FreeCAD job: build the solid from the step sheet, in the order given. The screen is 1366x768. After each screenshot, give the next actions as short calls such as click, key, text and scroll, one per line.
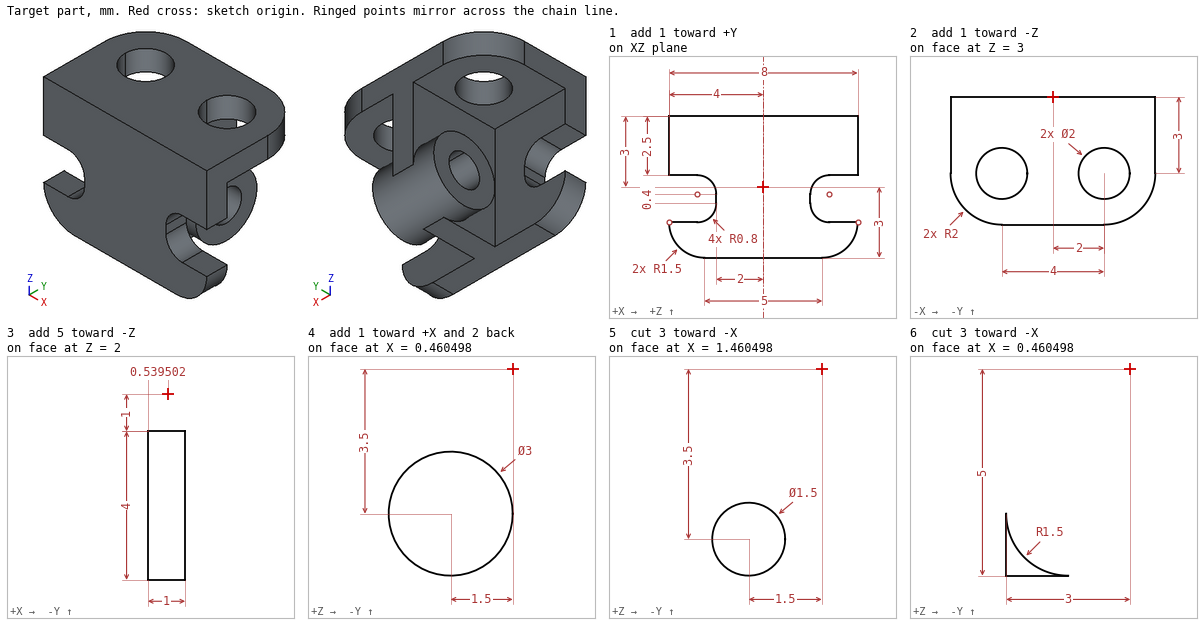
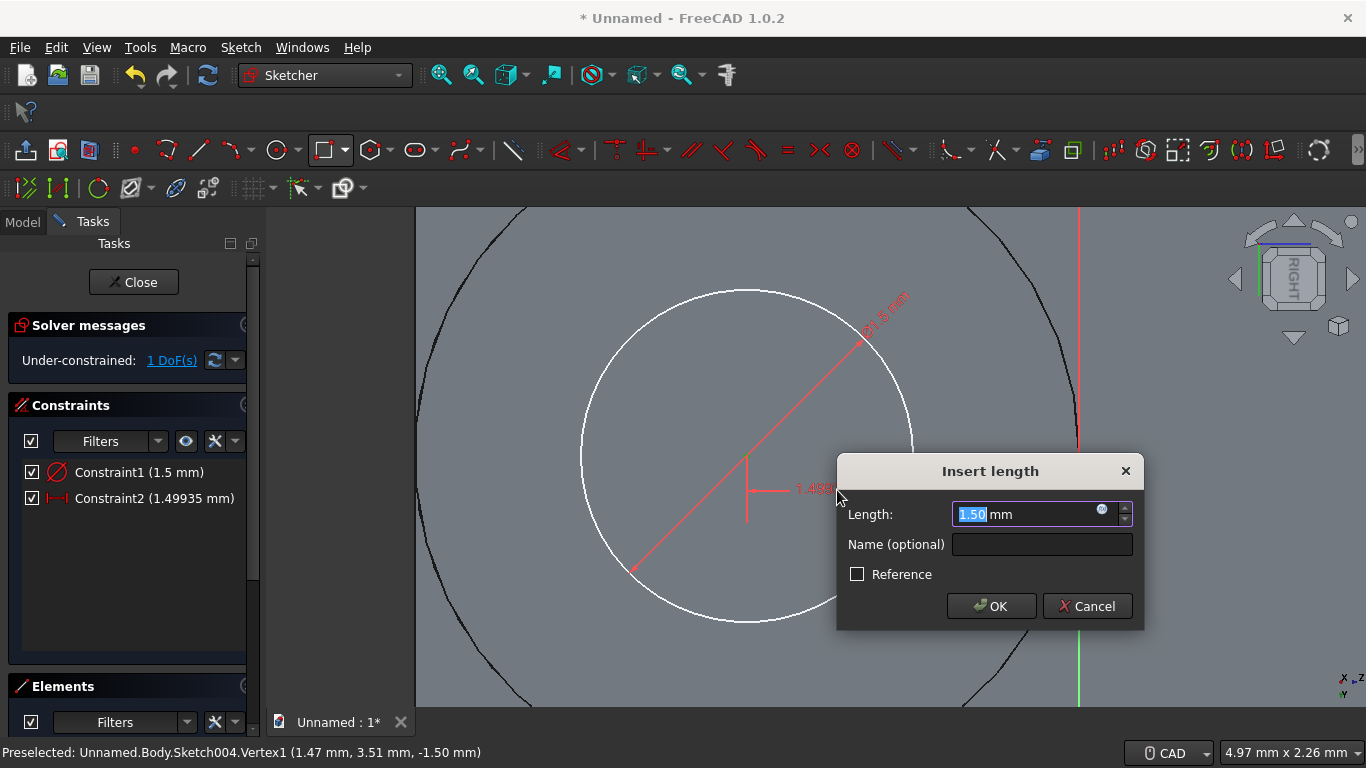
text(1.5)
key(Return)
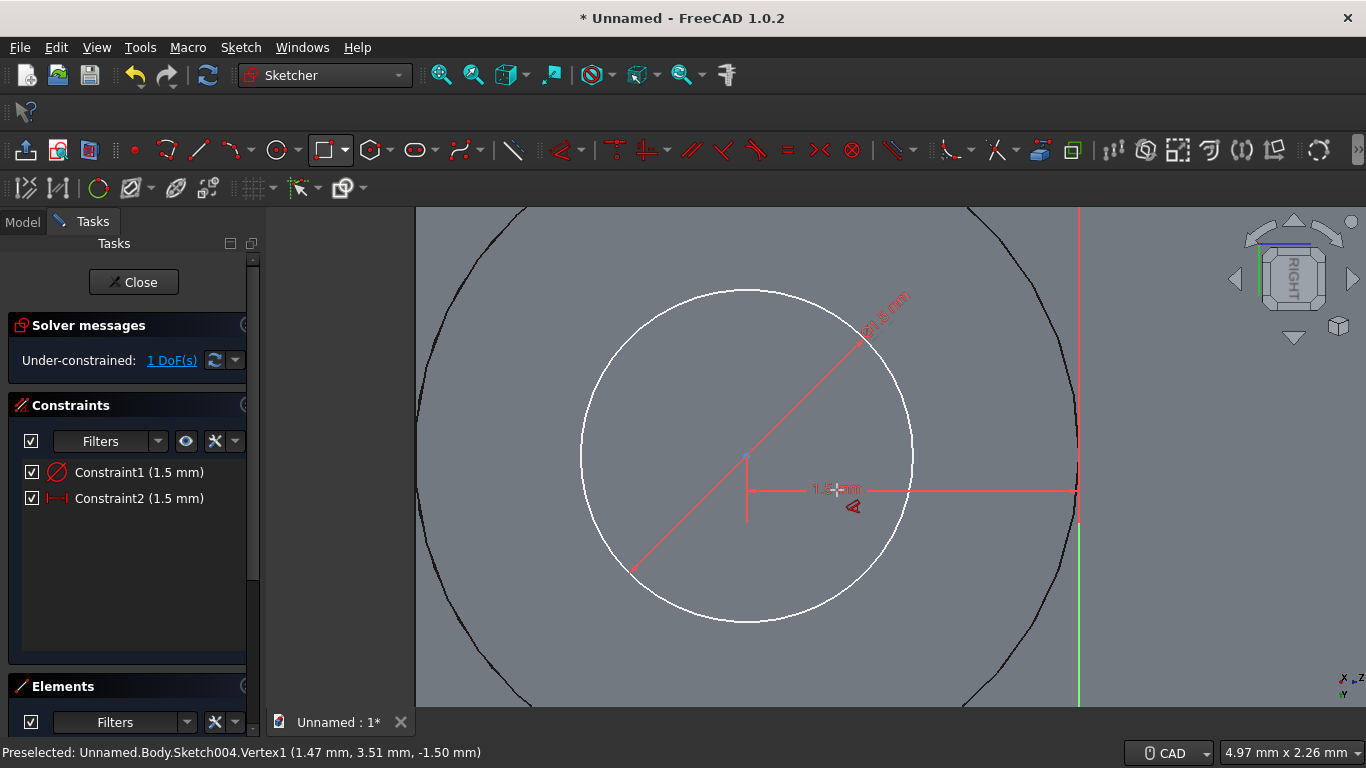
click(747, 456)
click(1113, 346)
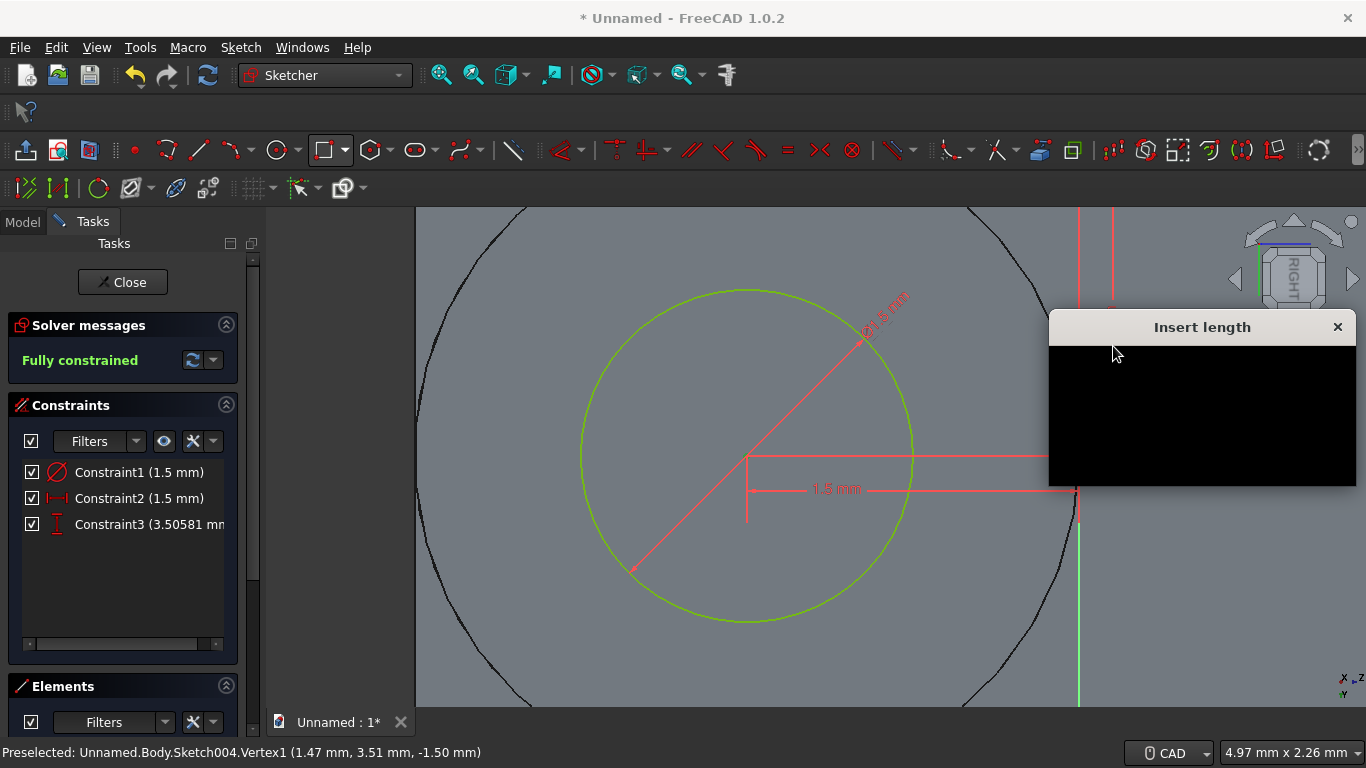
text(3.5)
key(Return)
key(Escape)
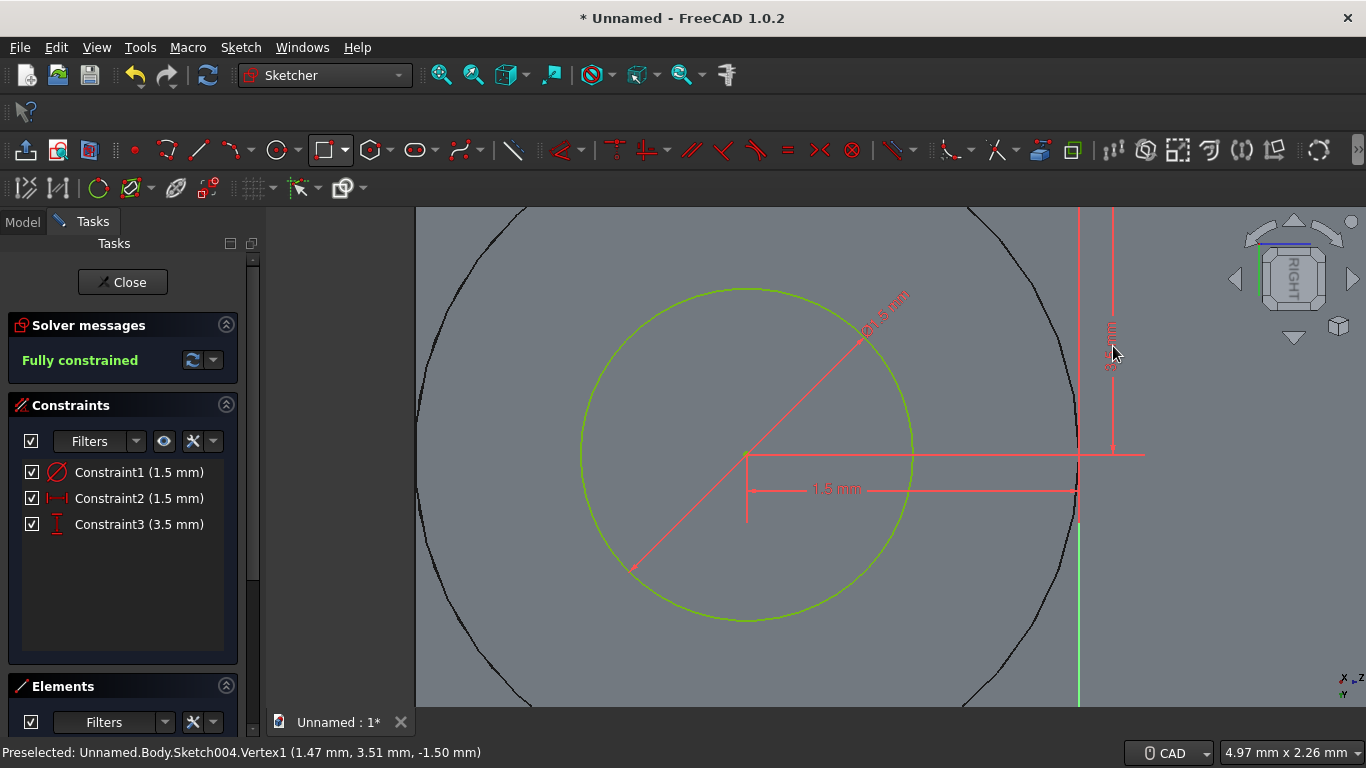
click(123, 282)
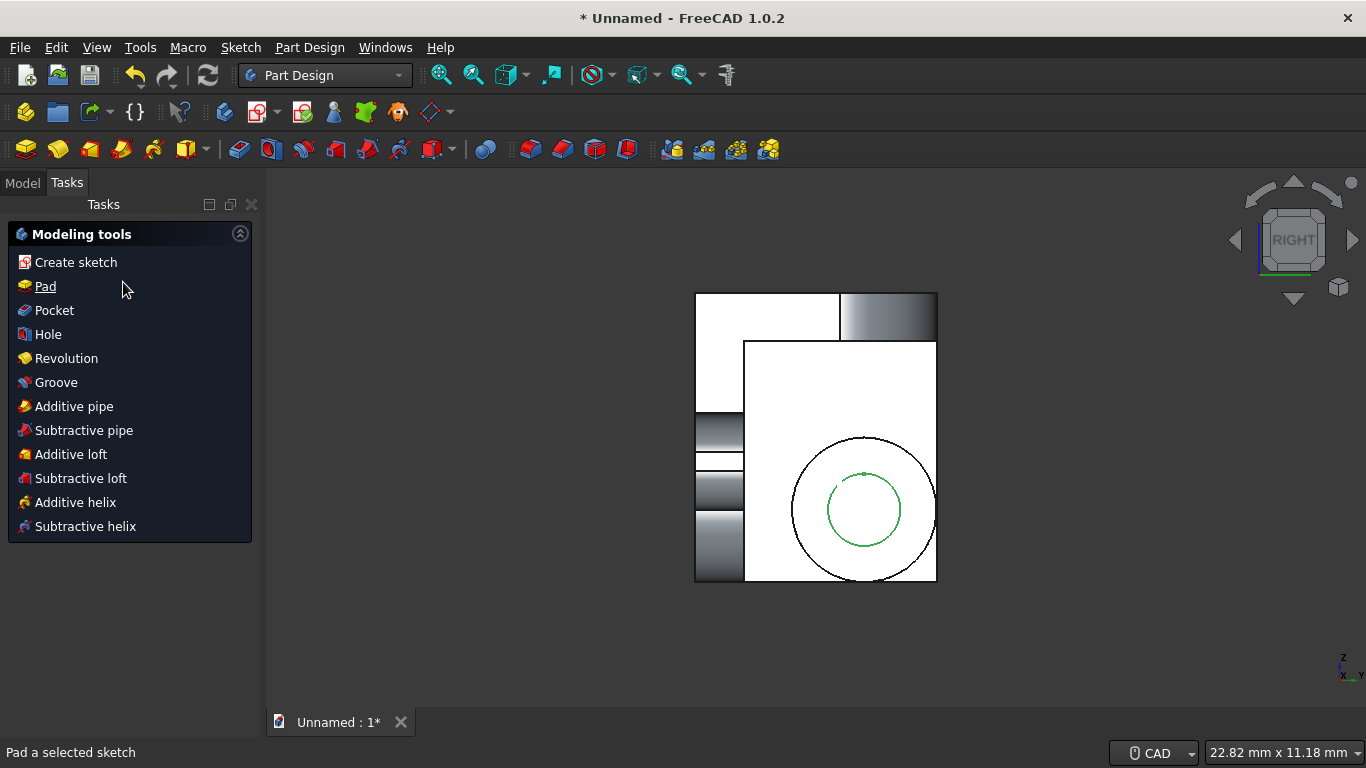
click(240, 150)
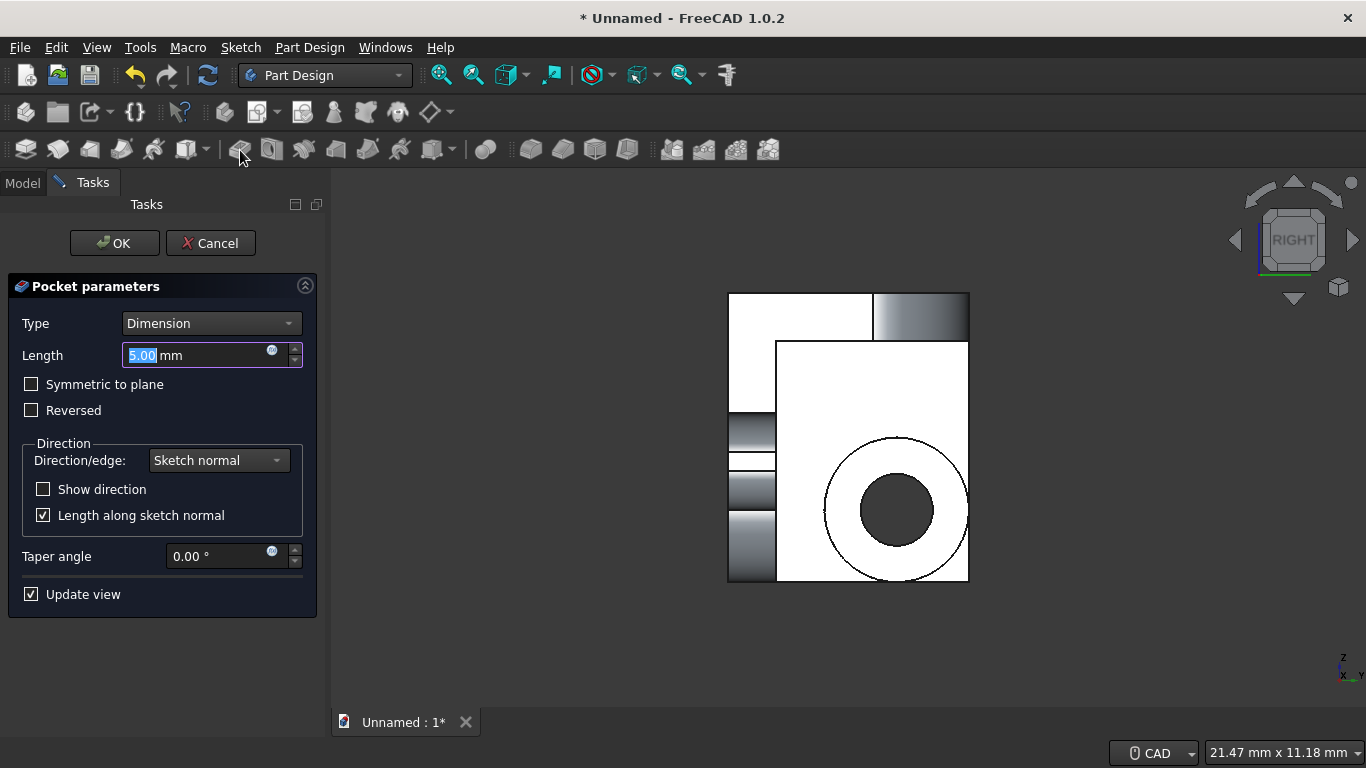
text(3)
key(Tab)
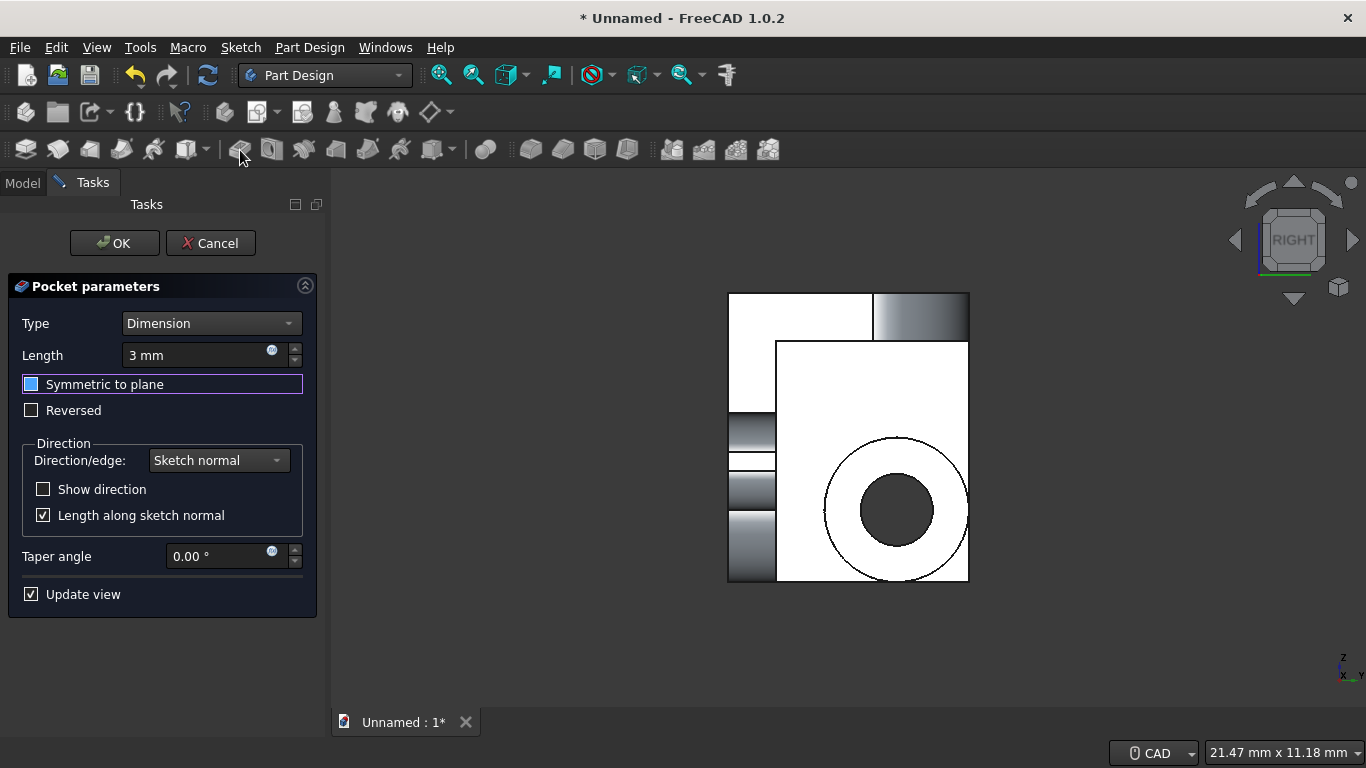
click(115, 243)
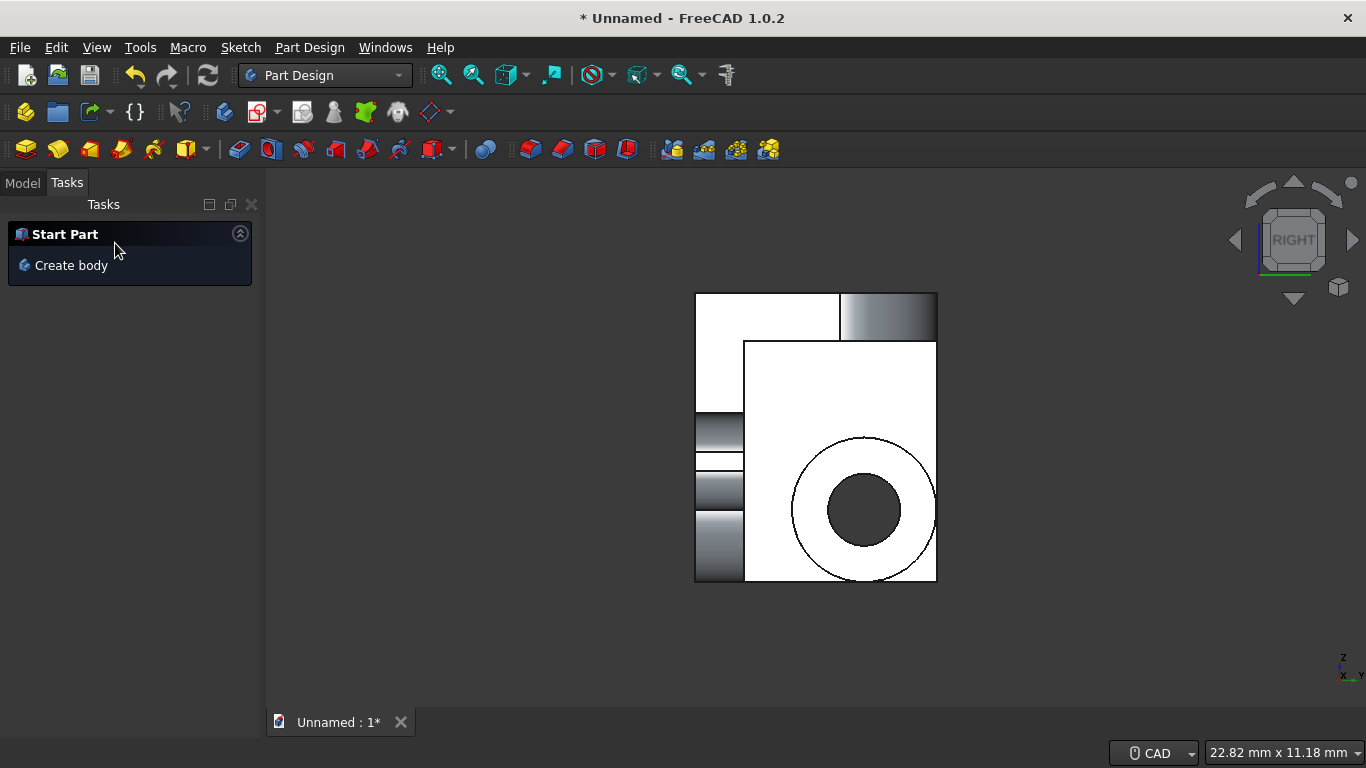
click(813, 392)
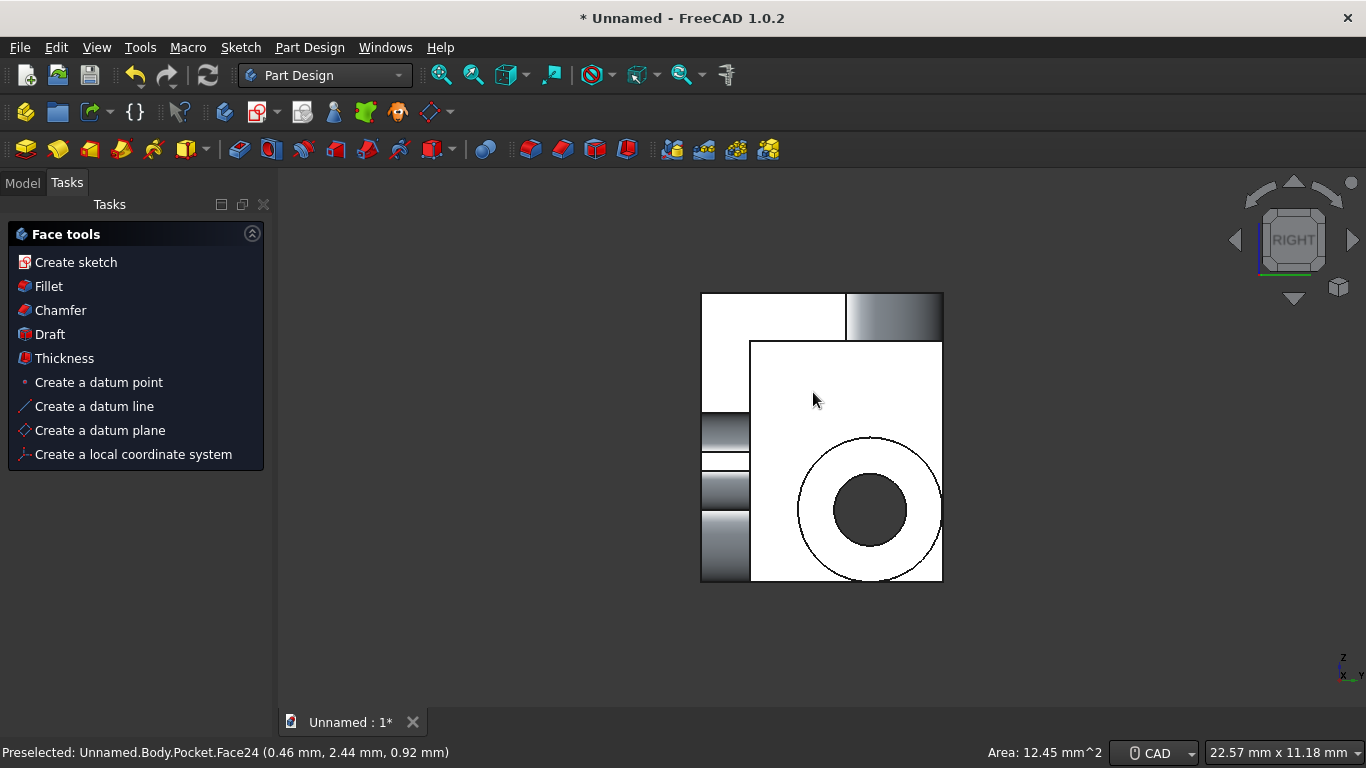
click(258, 112)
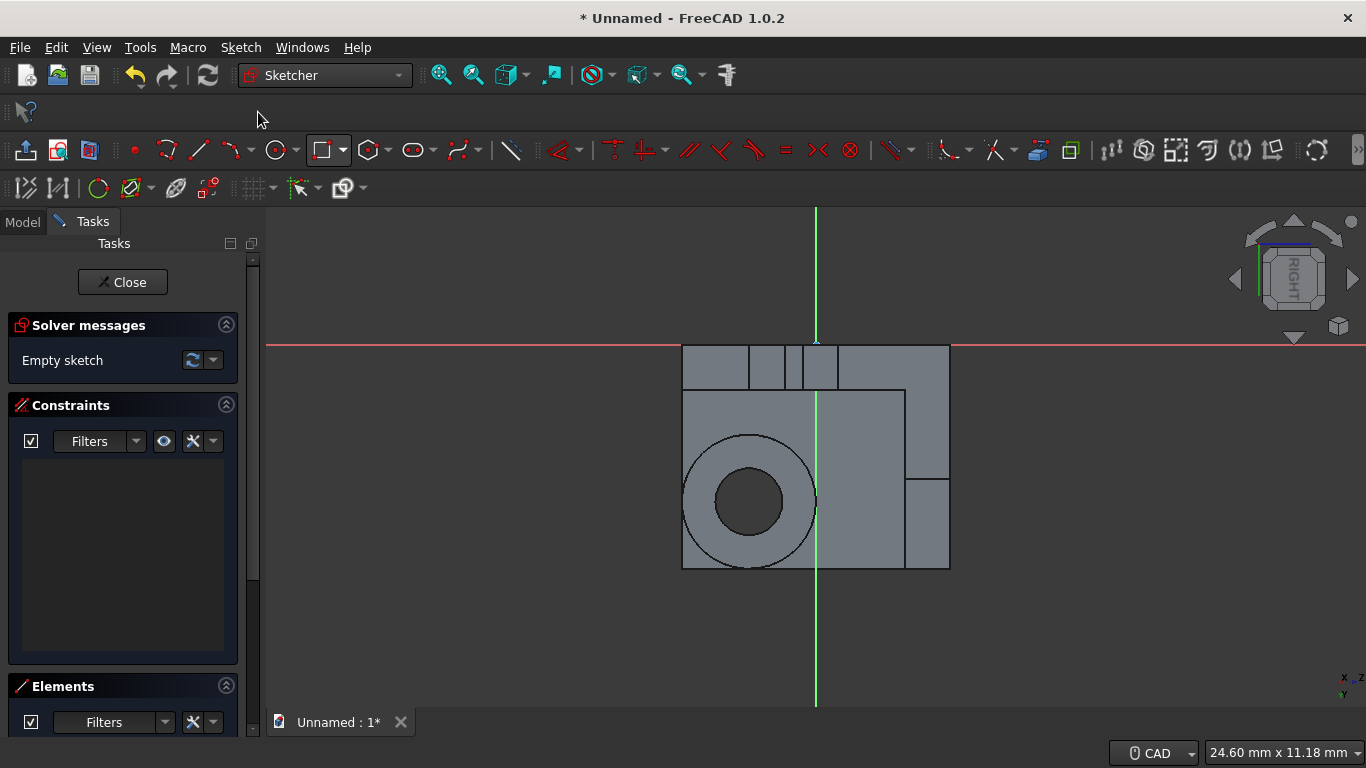
scroll(707, 555, up, 8)